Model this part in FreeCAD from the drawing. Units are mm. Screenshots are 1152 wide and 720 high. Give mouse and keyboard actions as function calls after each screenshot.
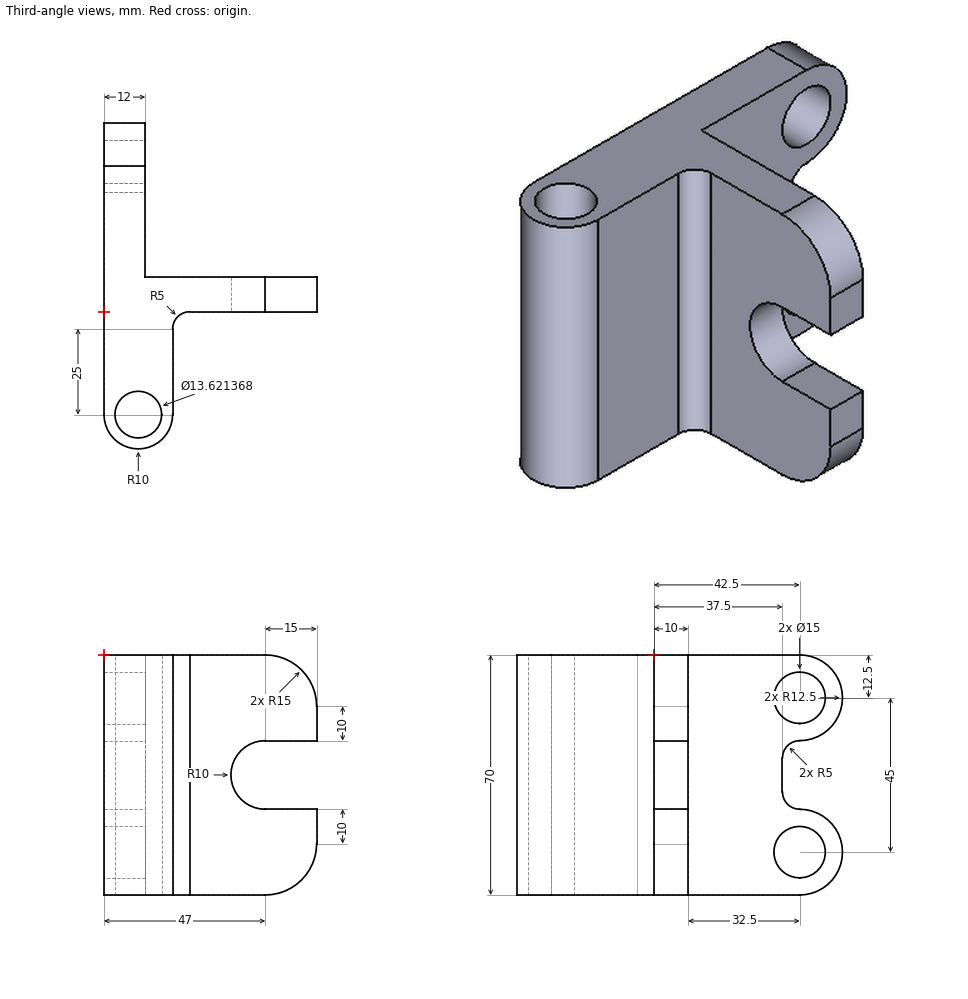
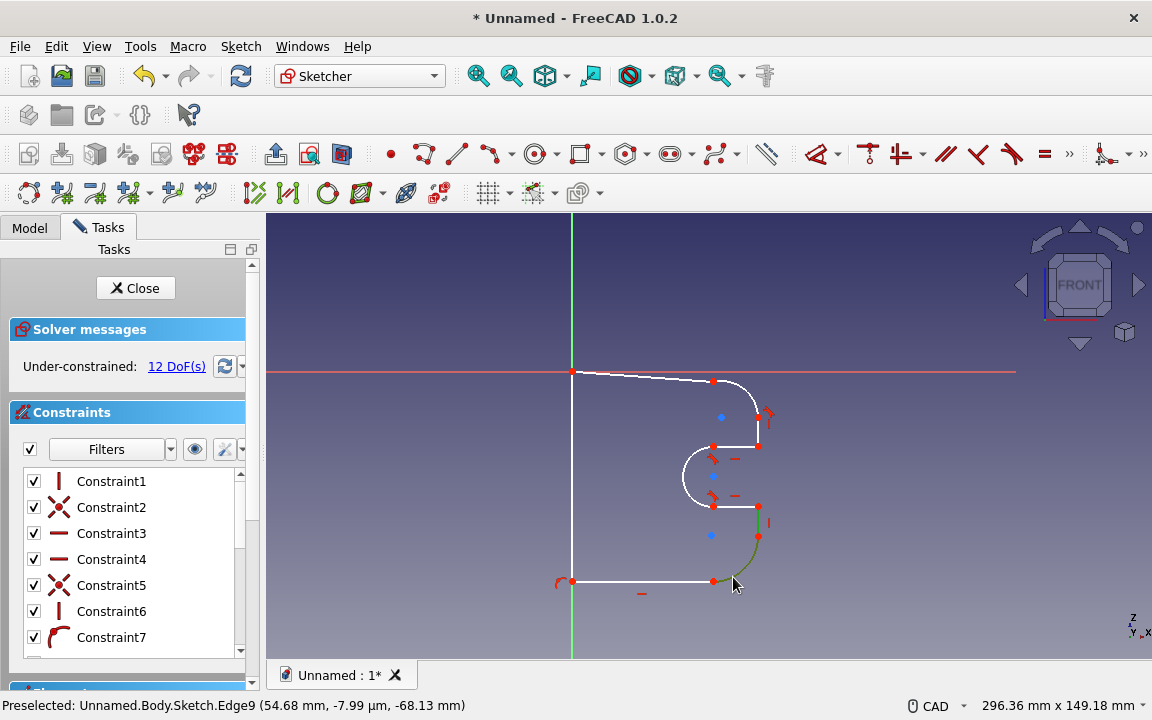
click(1012, 154)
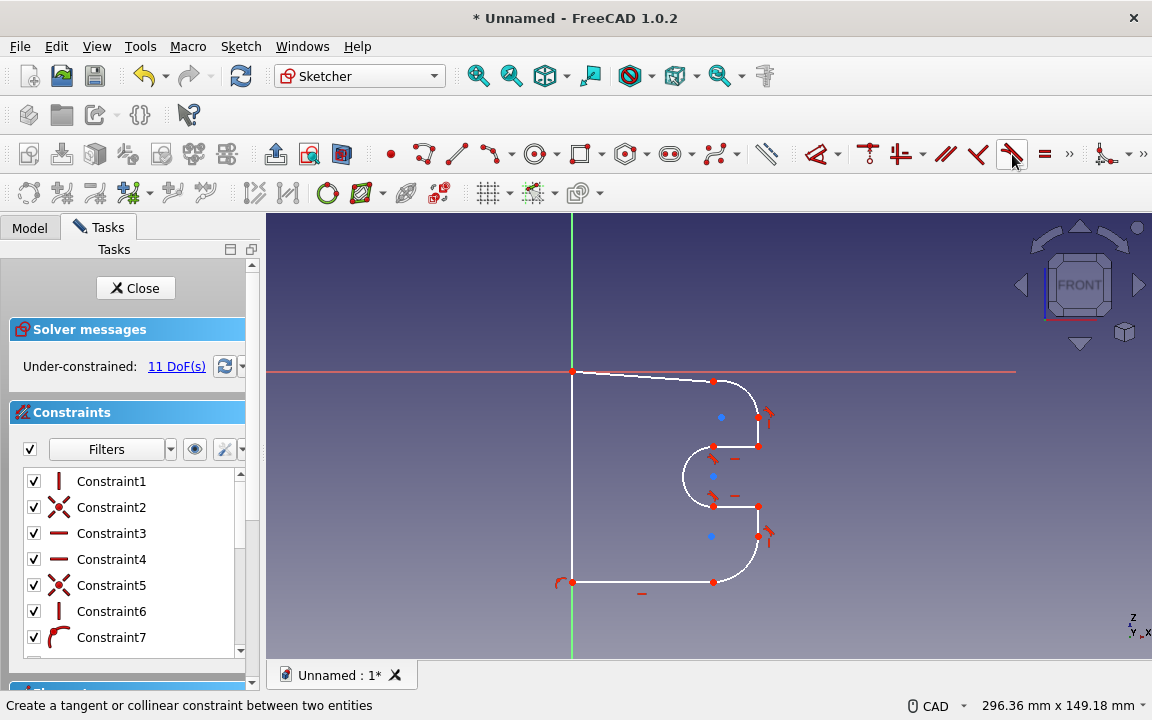
click(671, 582)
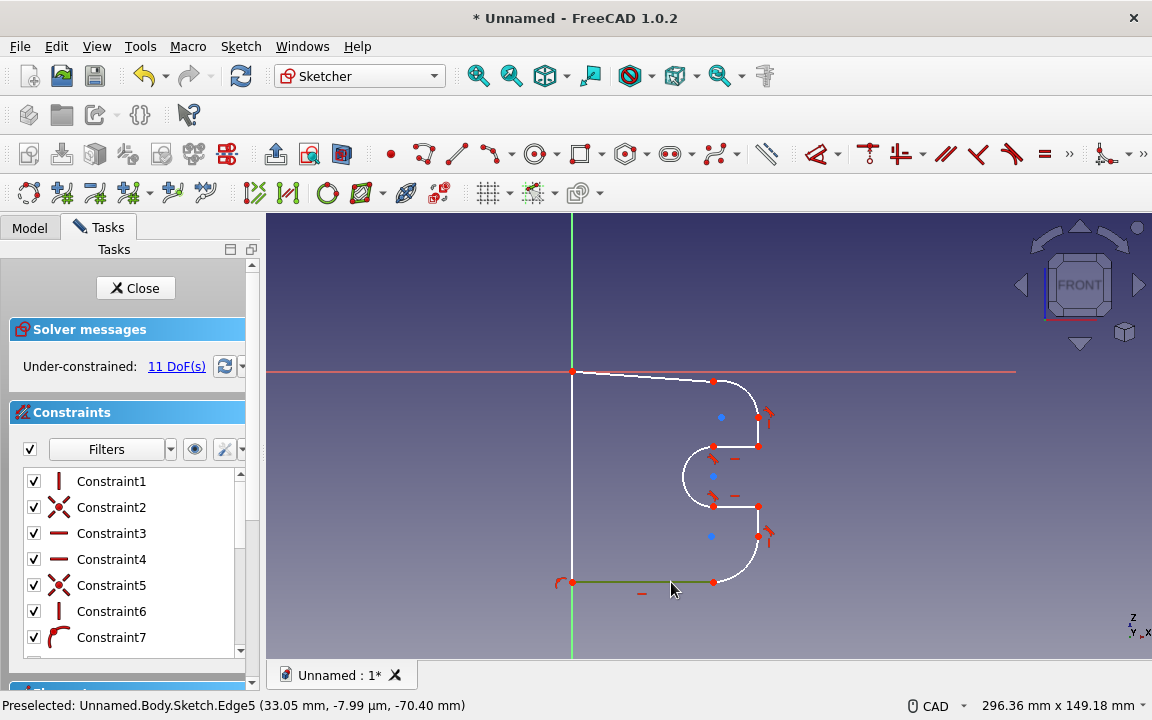
click(734, 577)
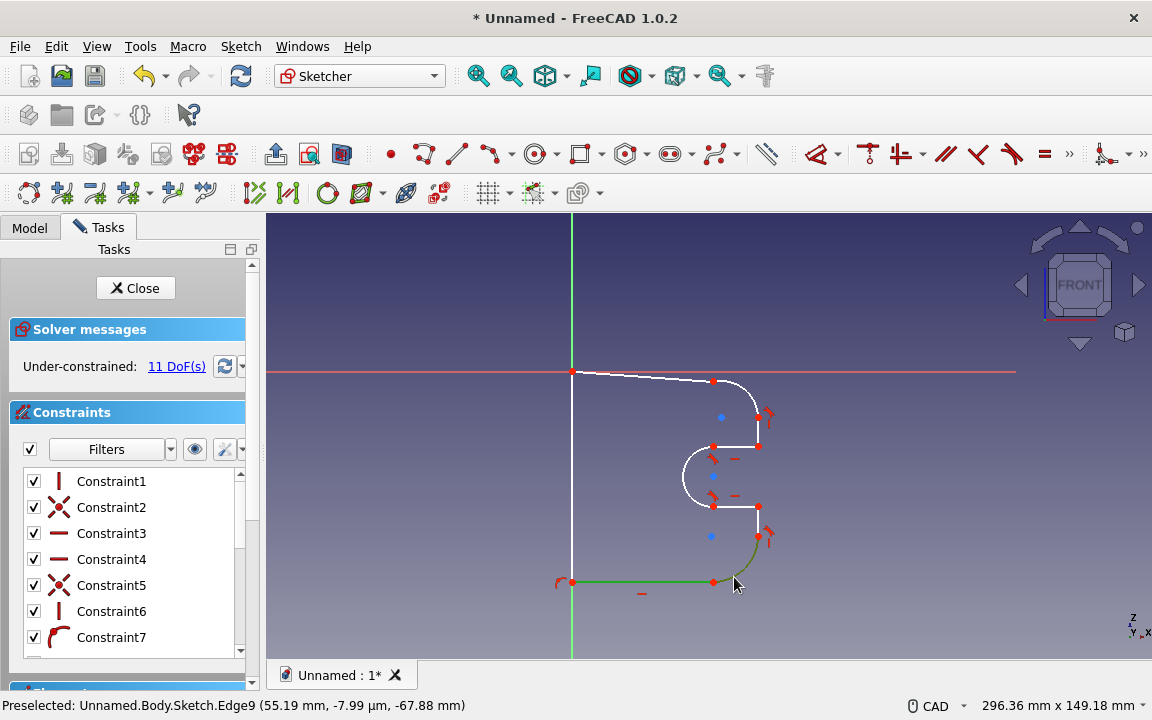
click(1012, 154)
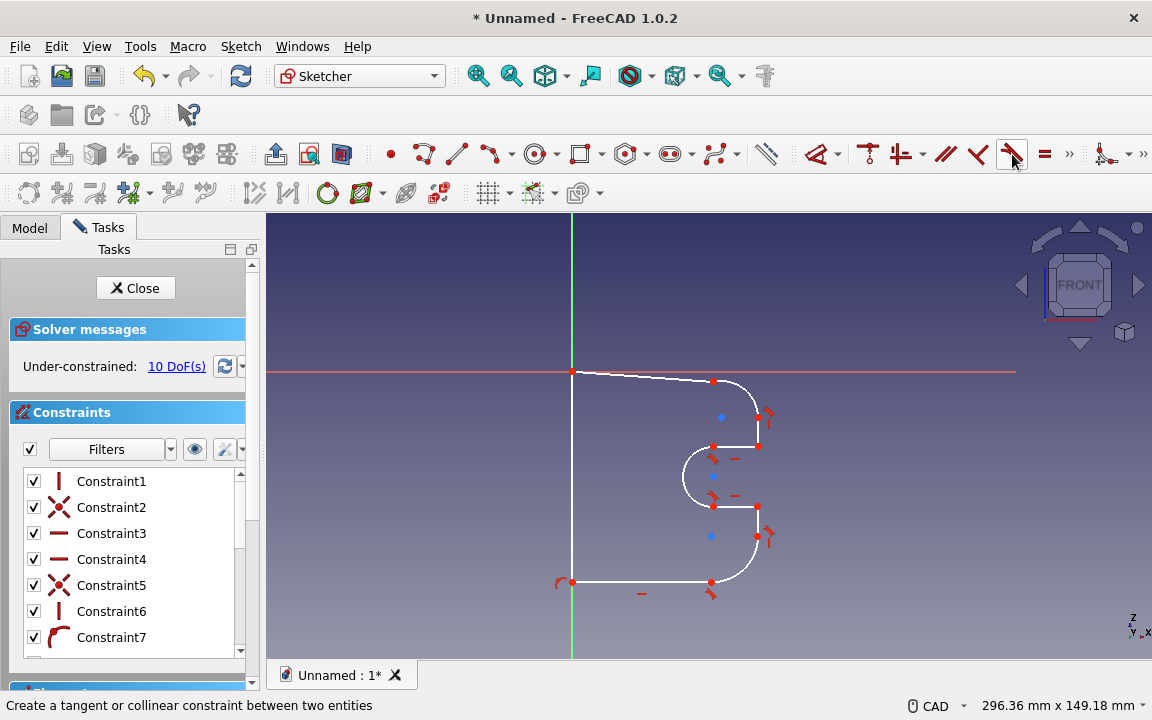
click(614, 375)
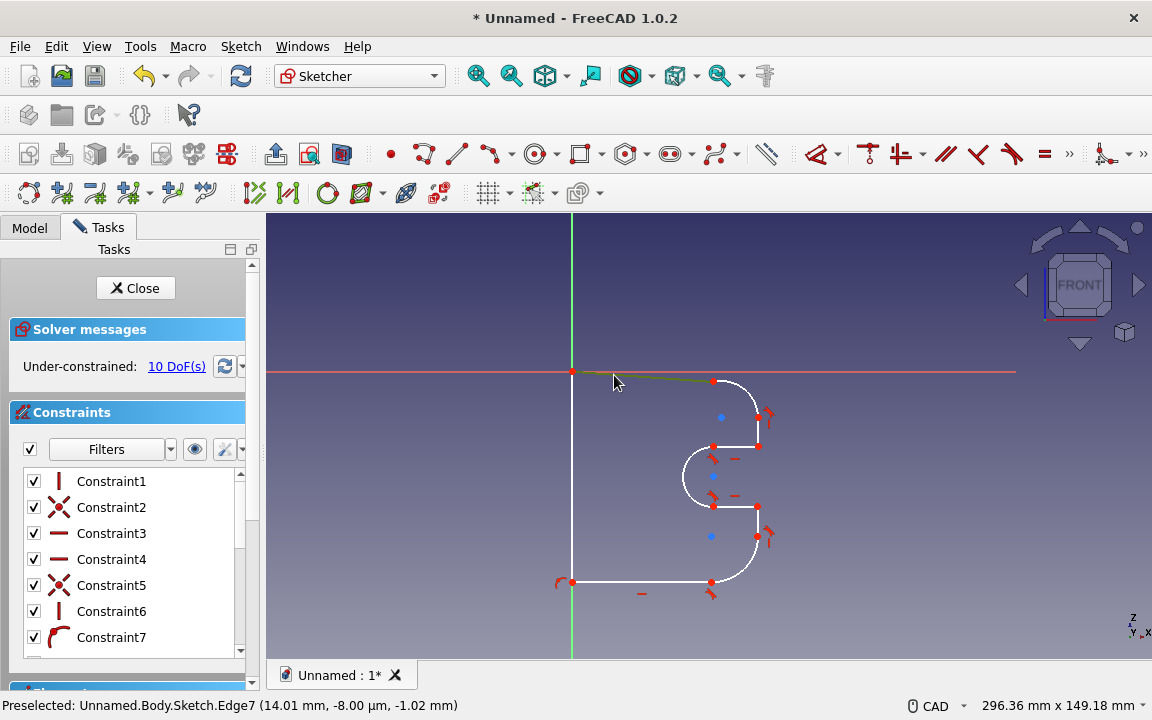
click(753, 399)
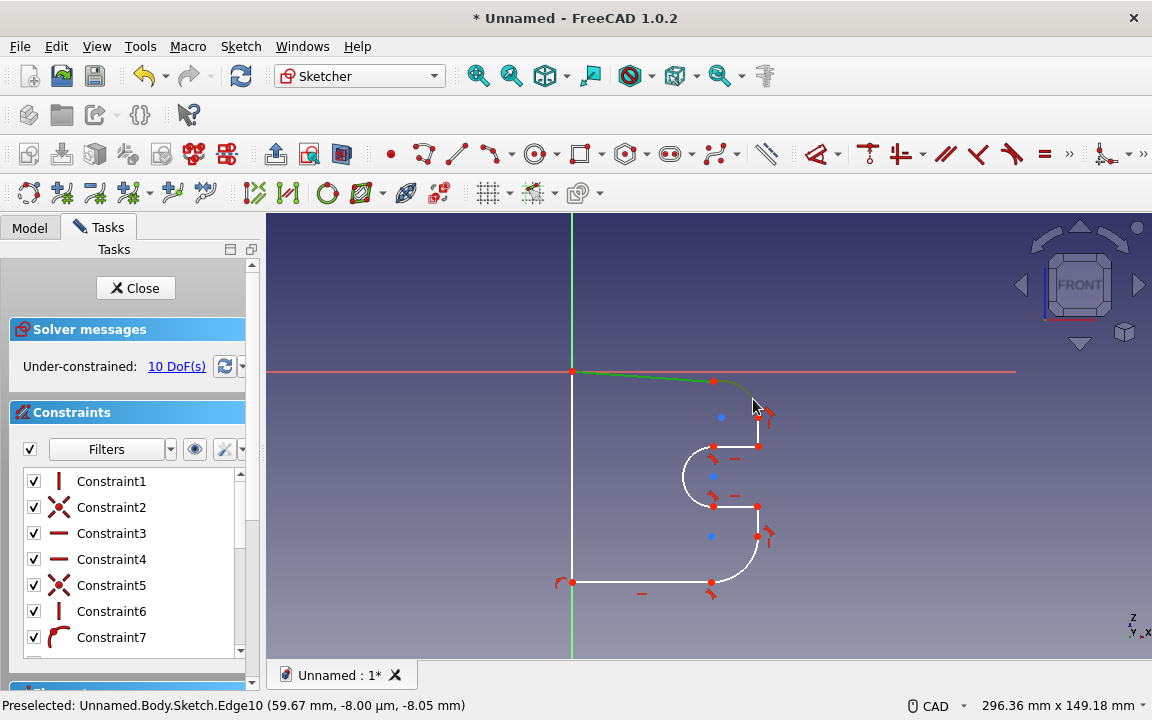
click(1012, 154)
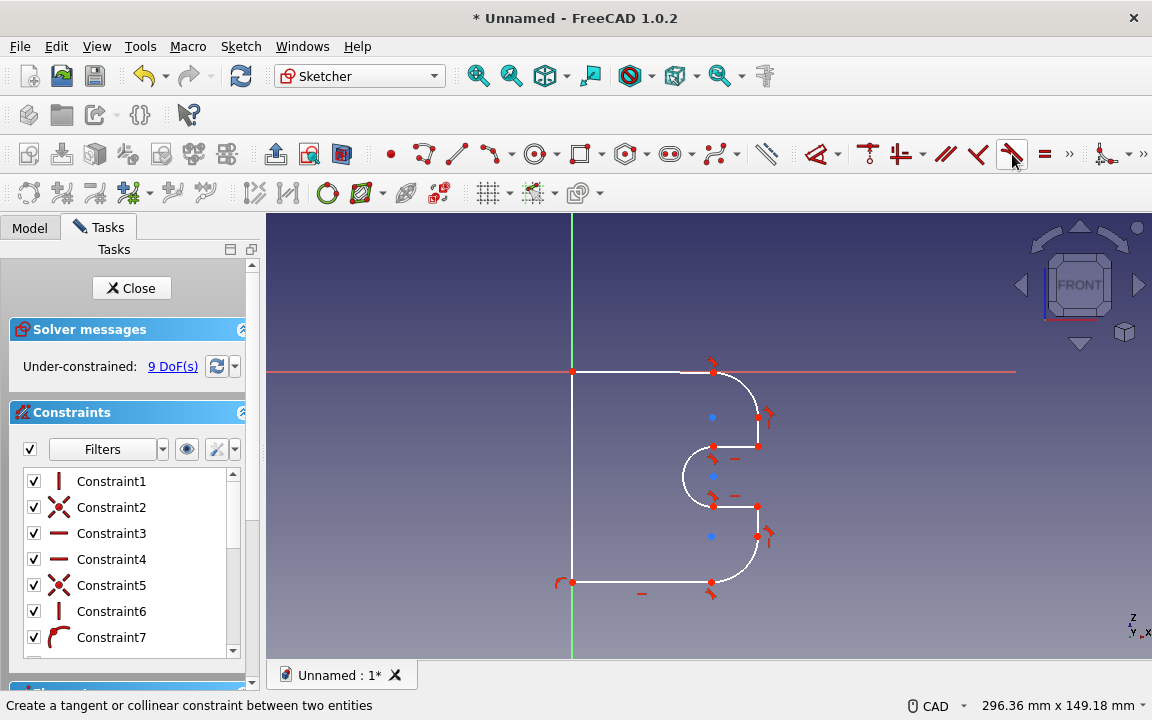
click(614, 372)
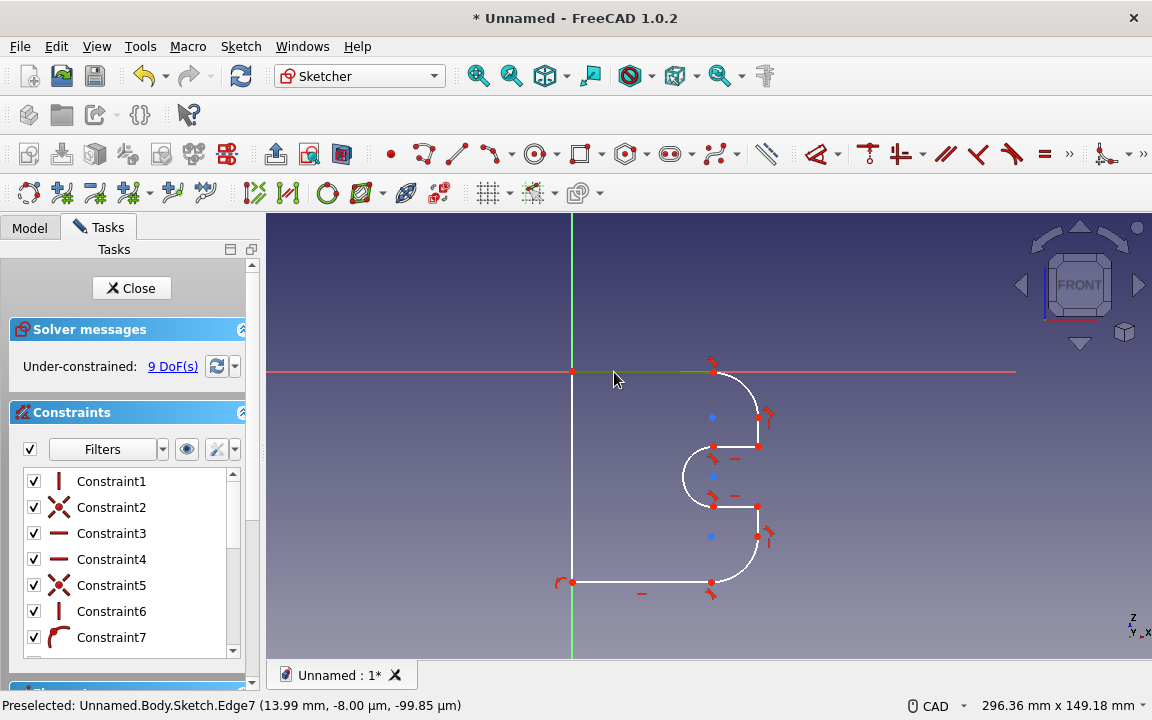
key(h)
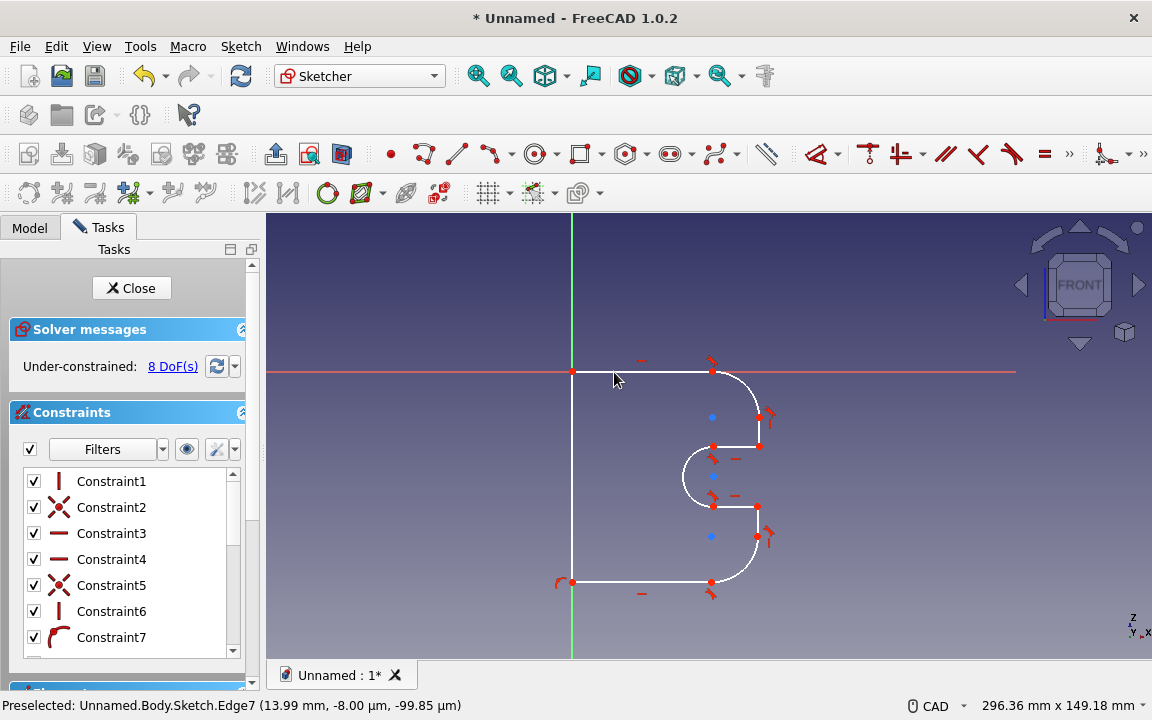
click(733, 577)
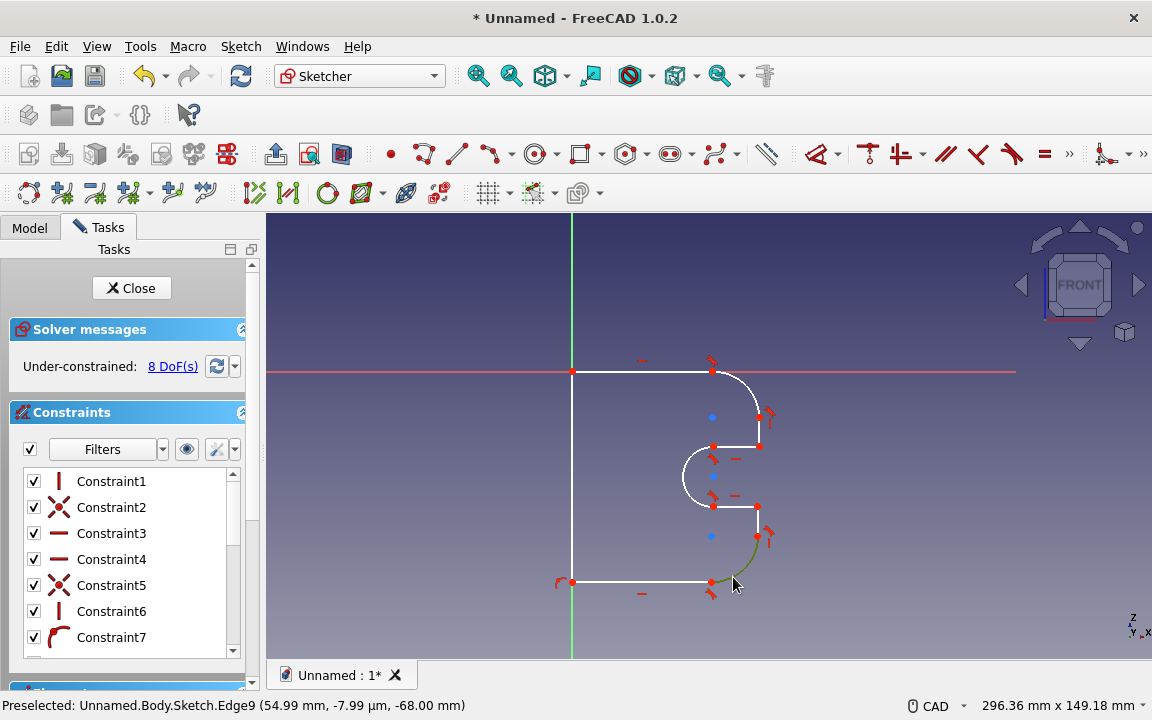
click(754, 397)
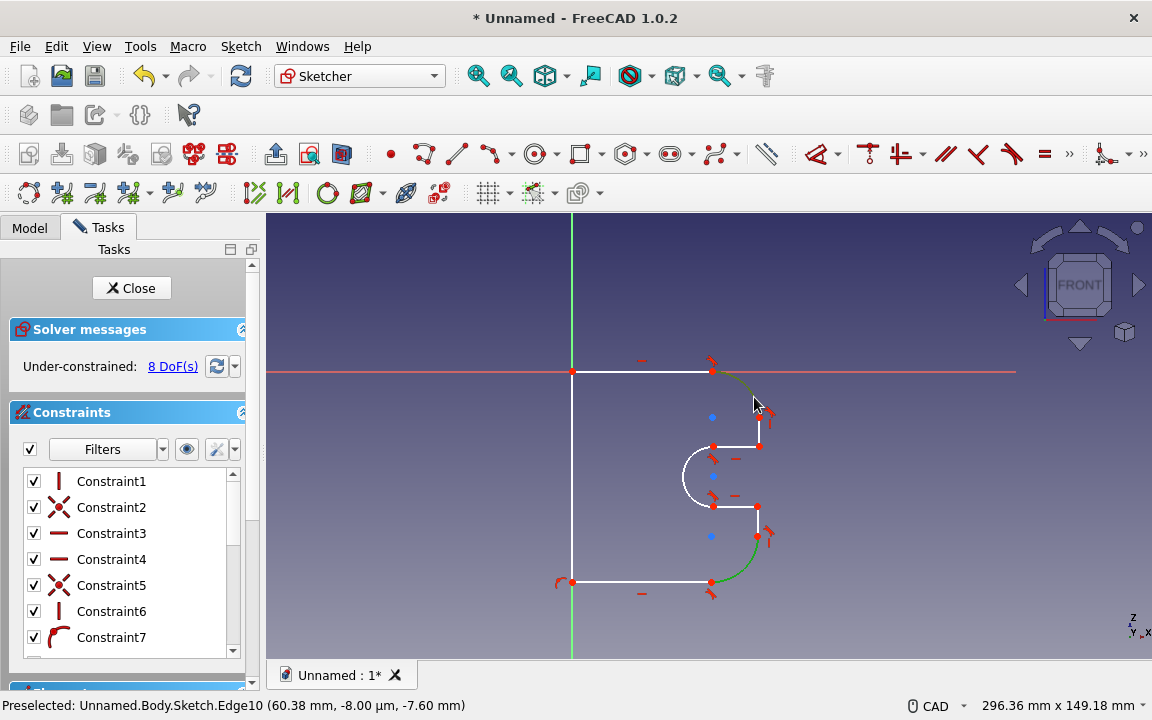
key(e)